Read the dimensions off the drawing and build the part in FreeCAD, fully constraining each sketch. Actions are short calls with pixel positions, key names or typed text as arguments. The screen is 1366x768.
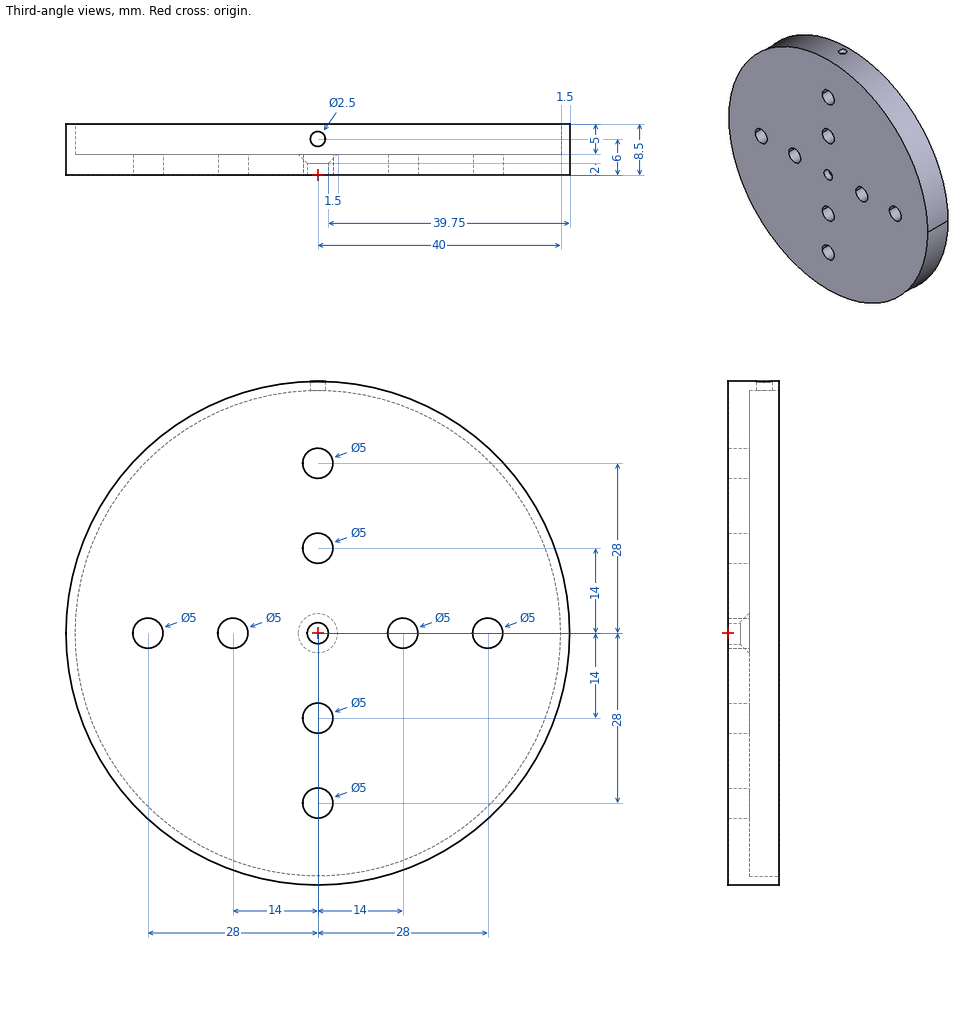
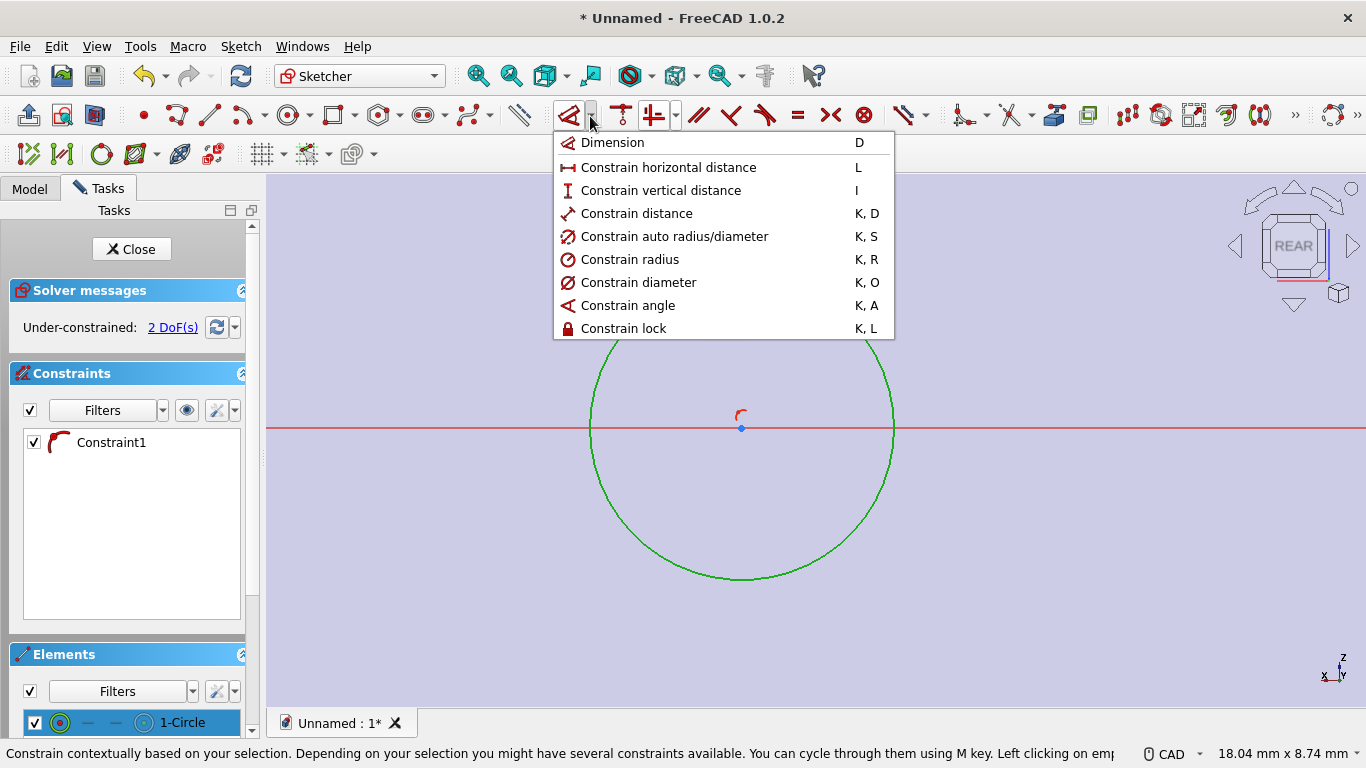
click(724, 282)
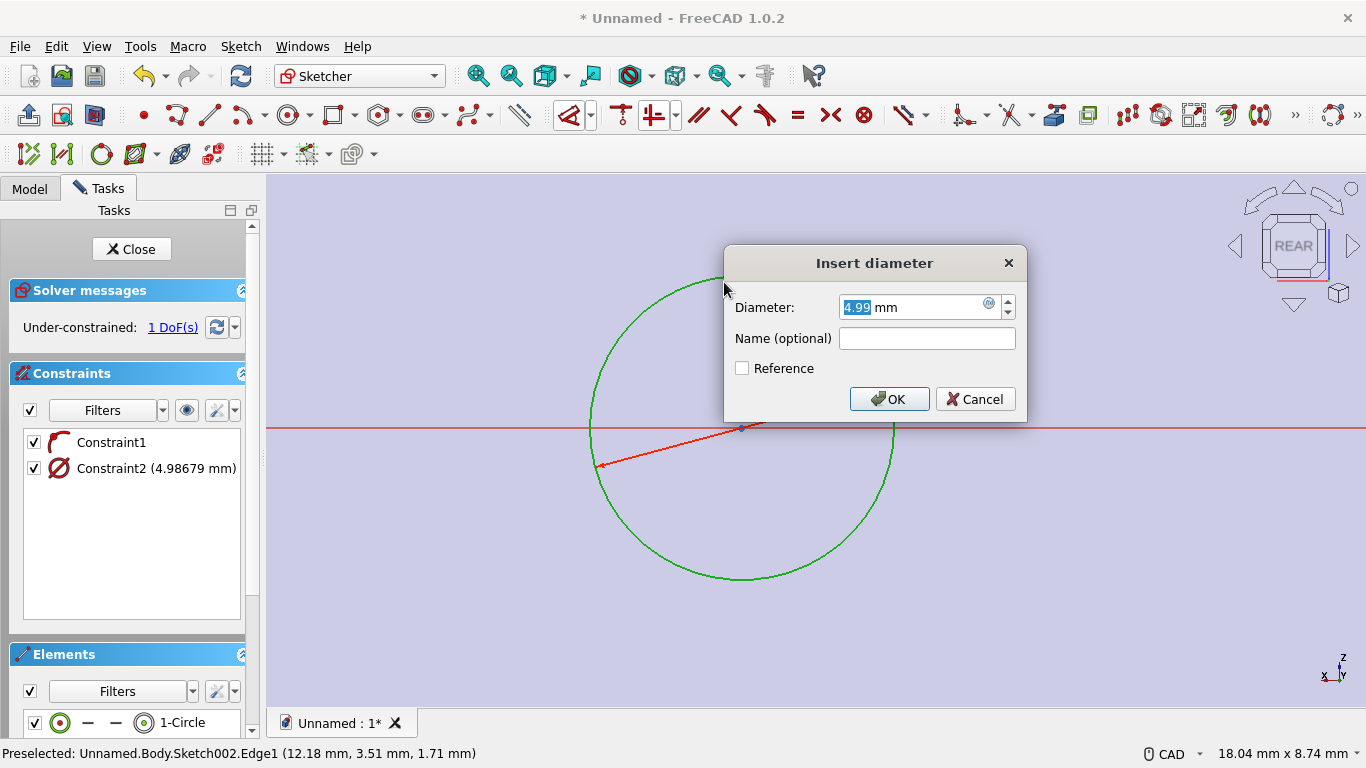
text(5)
key(Return)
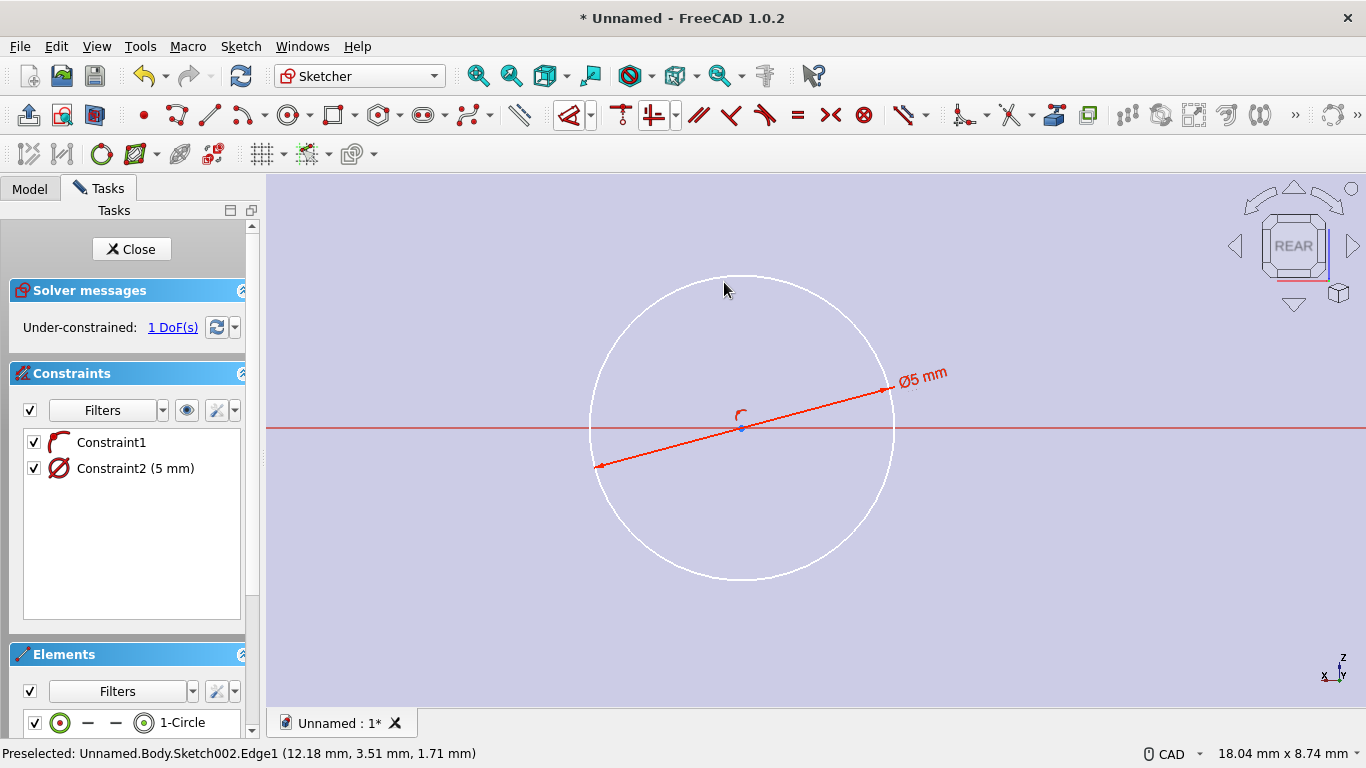
click(742, 428)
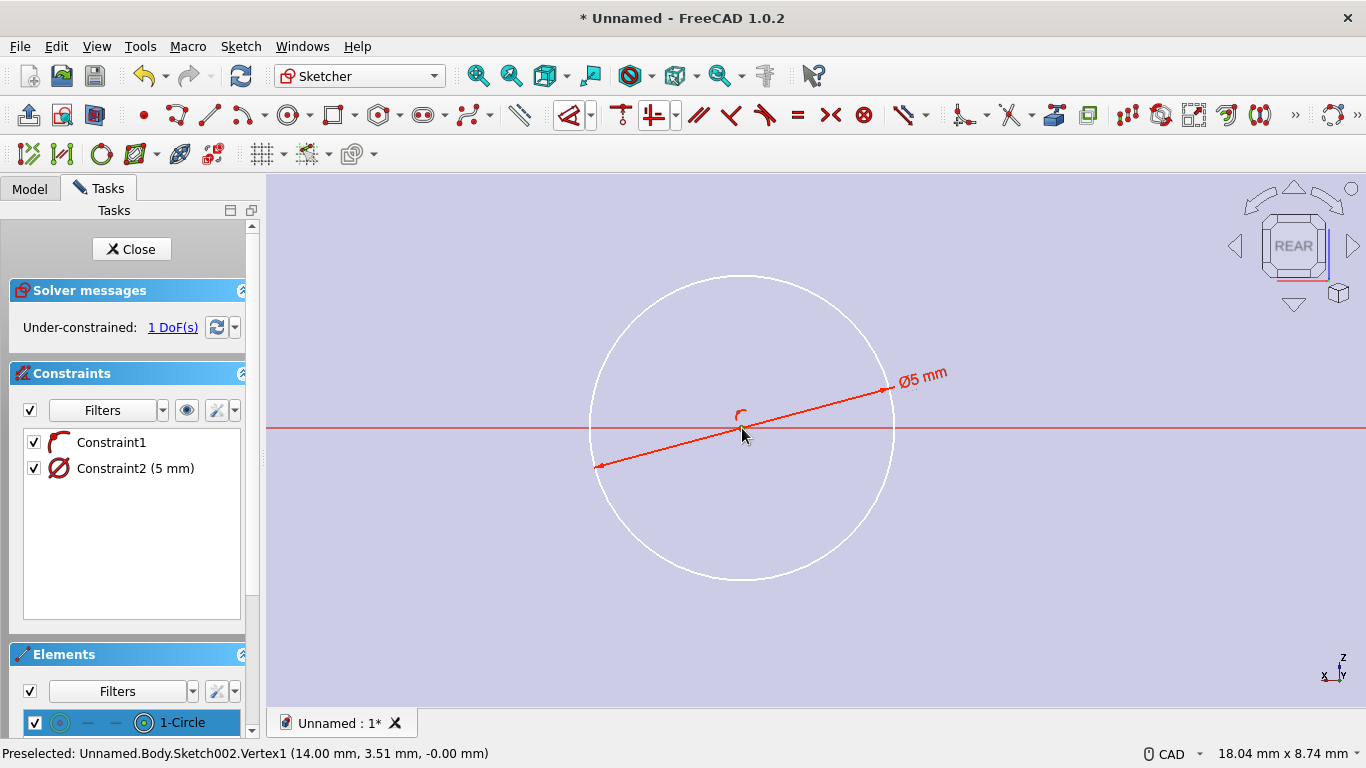
key(l)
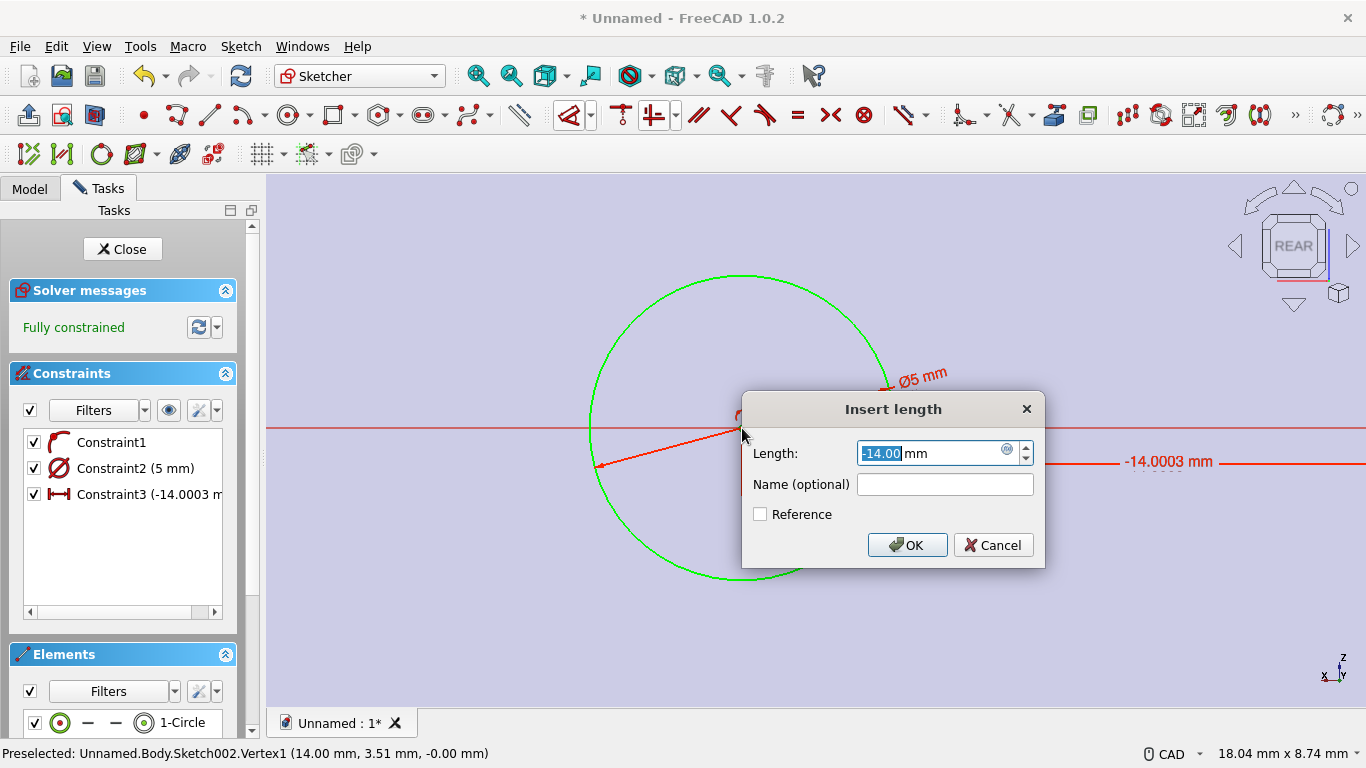
text(-14)
key(Return)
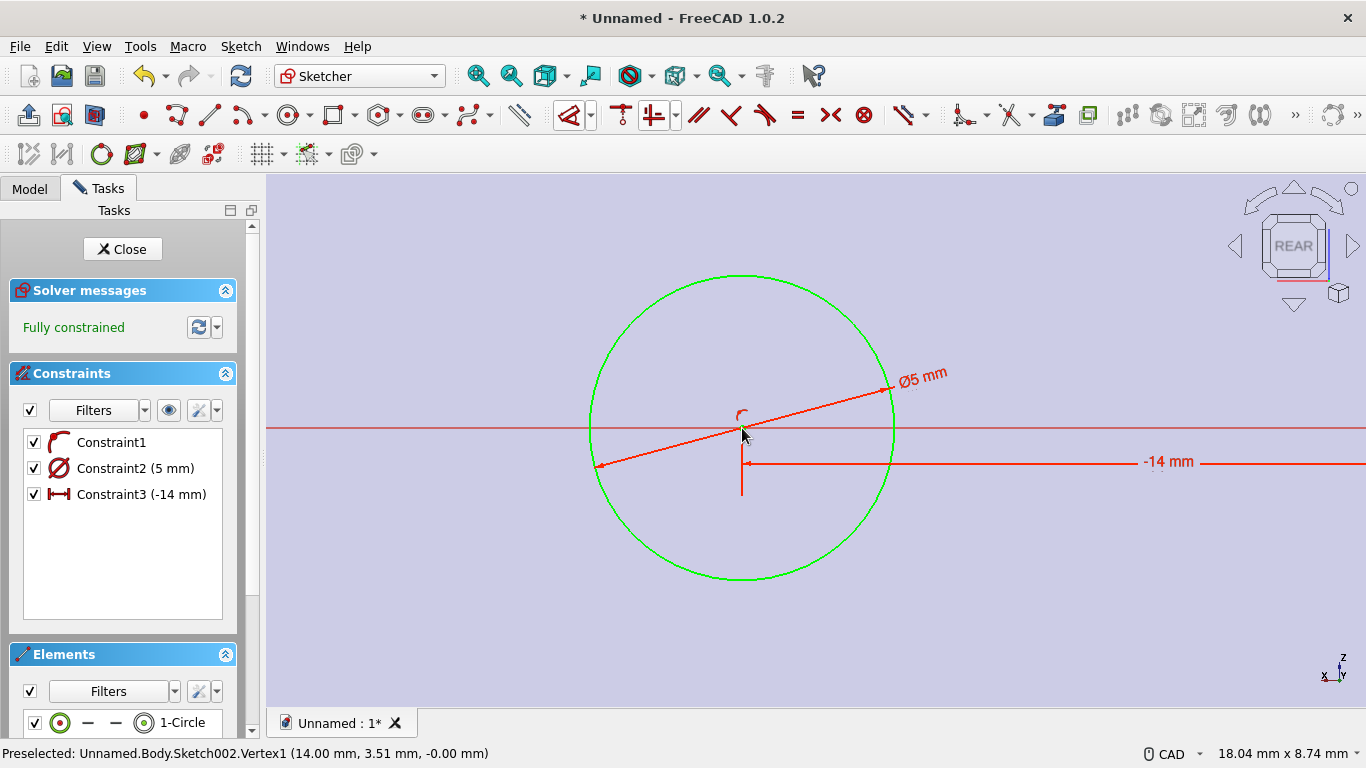
click(123, 249)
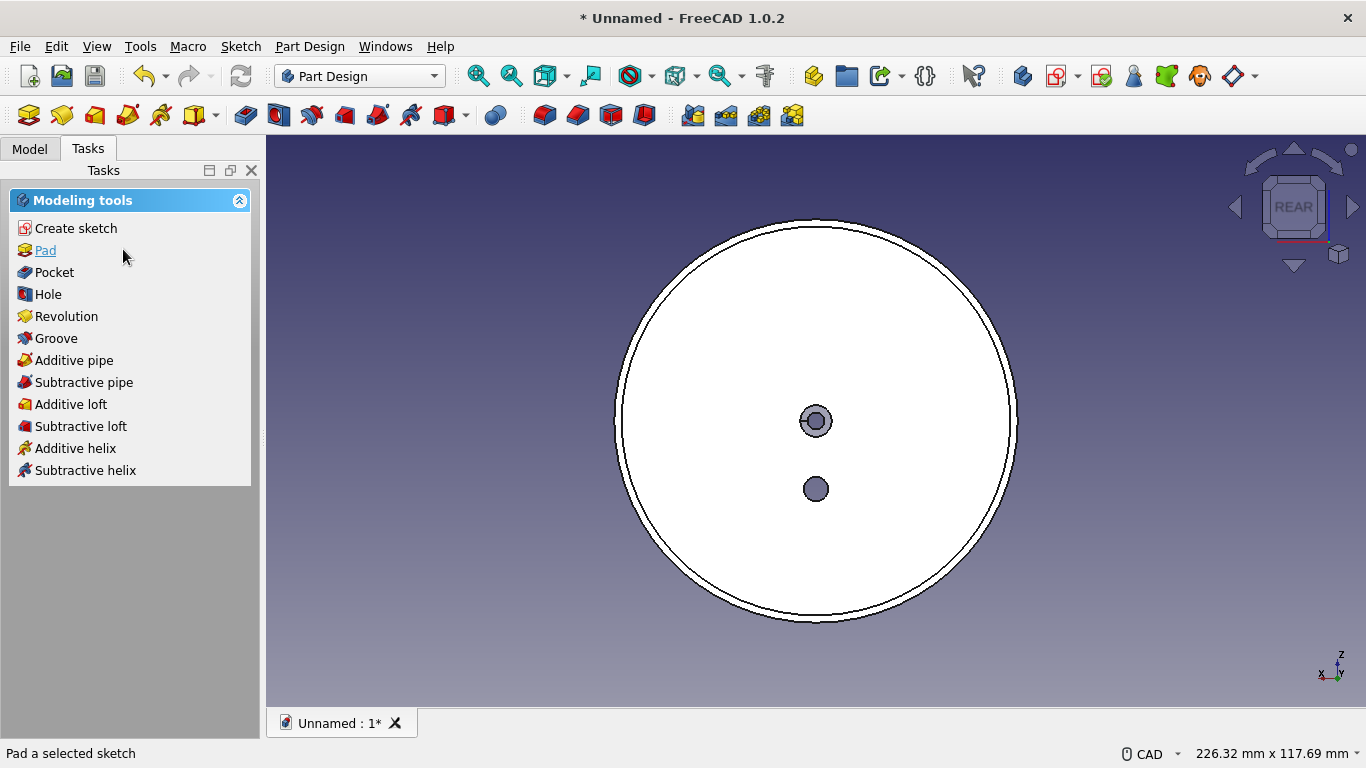
click(246, 116)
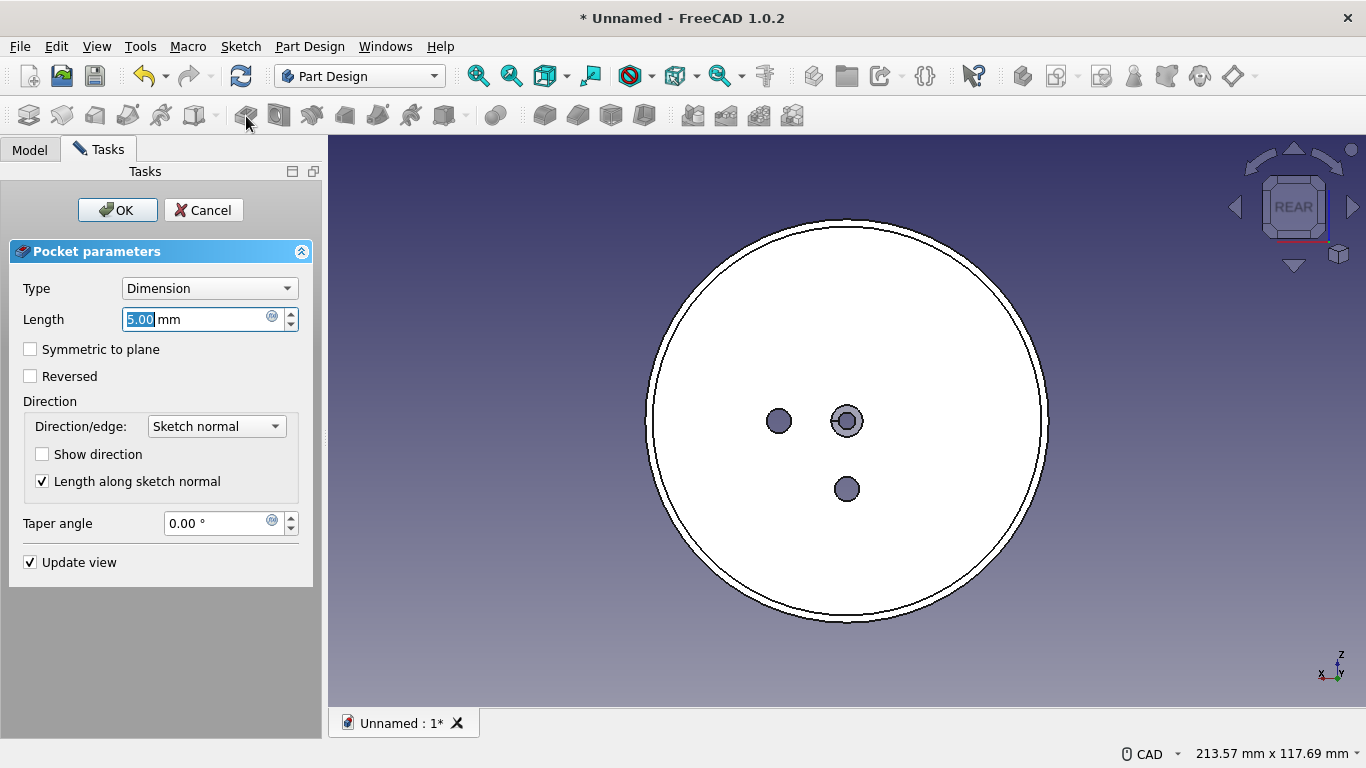
click(210, 288)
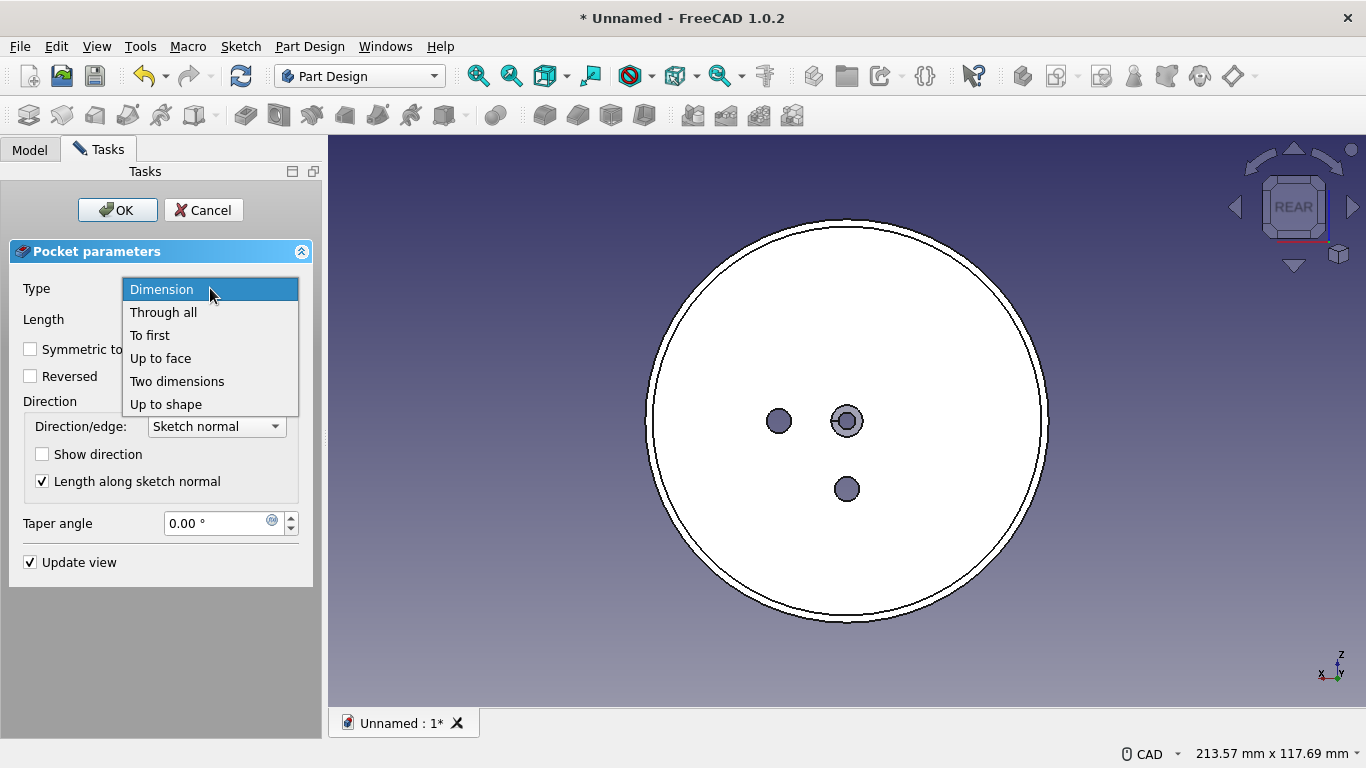
click(208, 336)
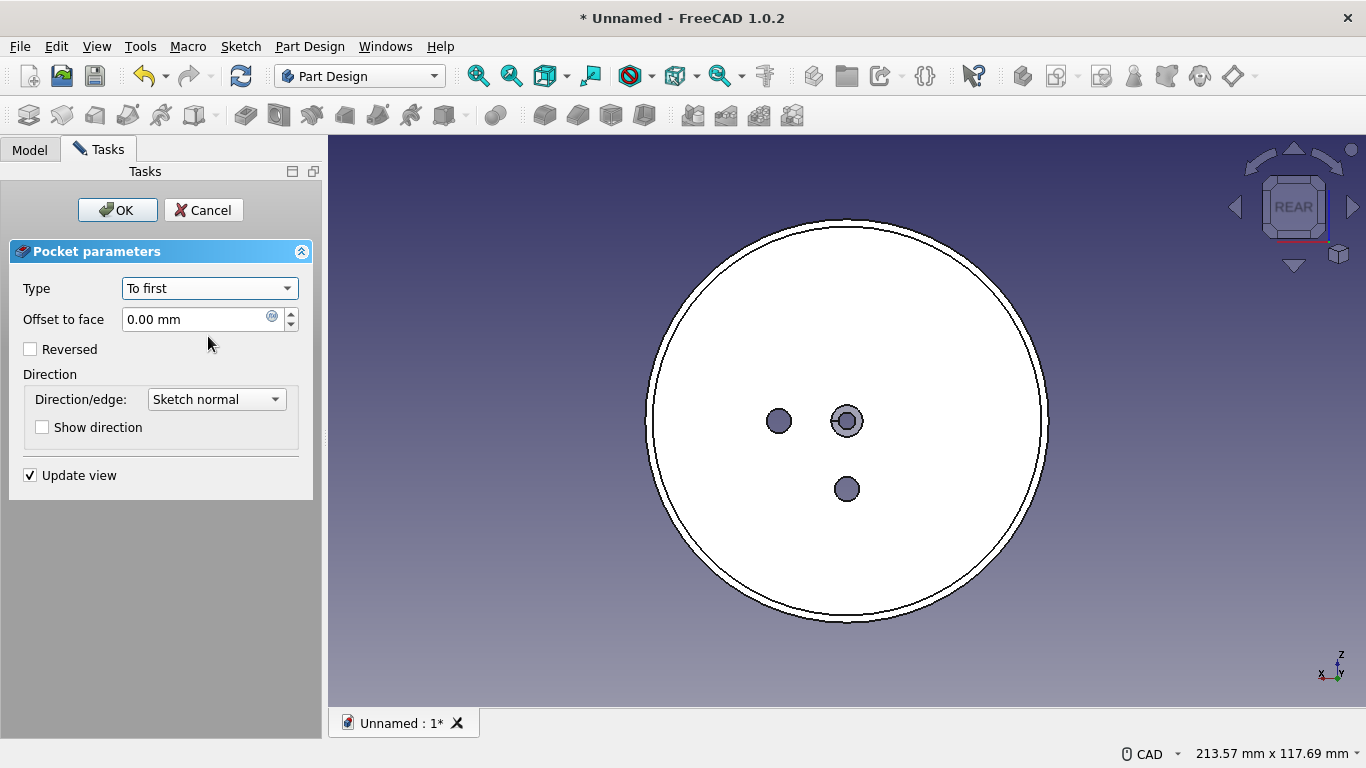
click(118, 210)